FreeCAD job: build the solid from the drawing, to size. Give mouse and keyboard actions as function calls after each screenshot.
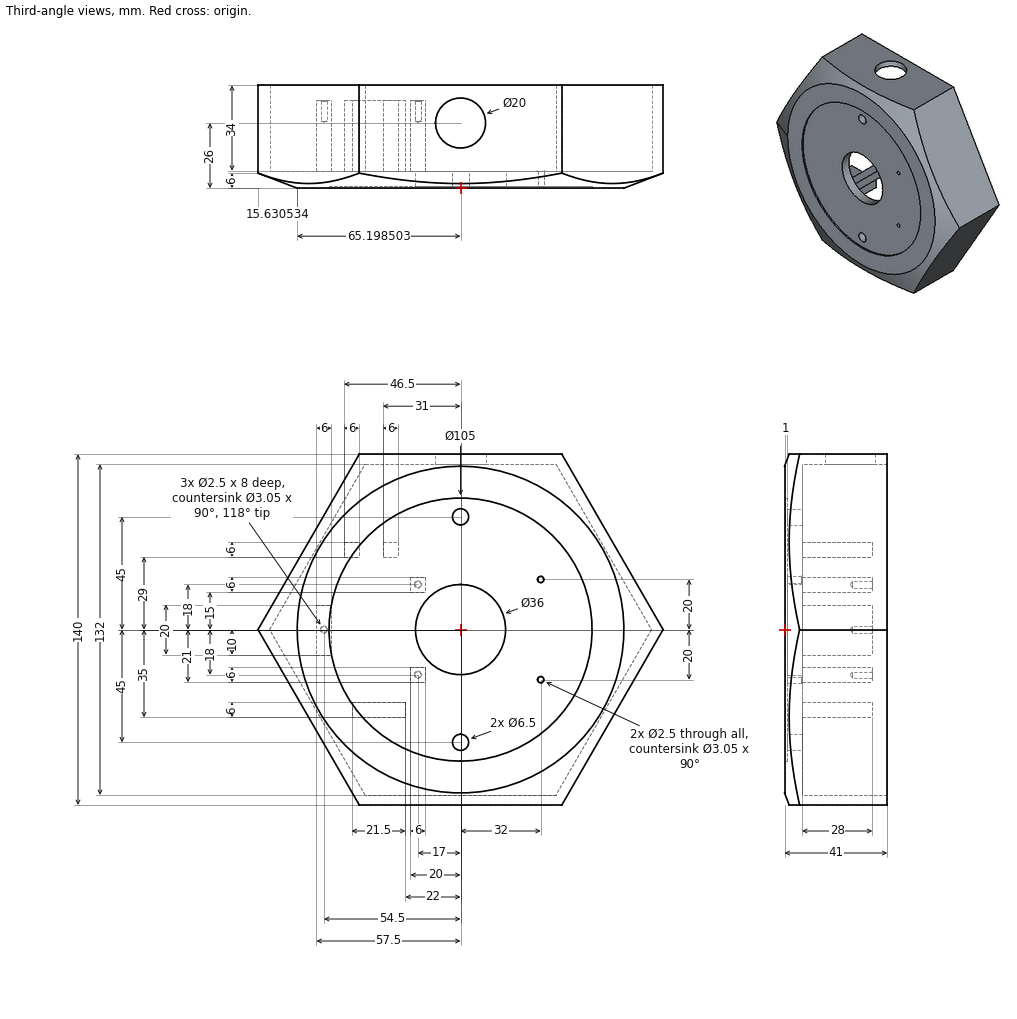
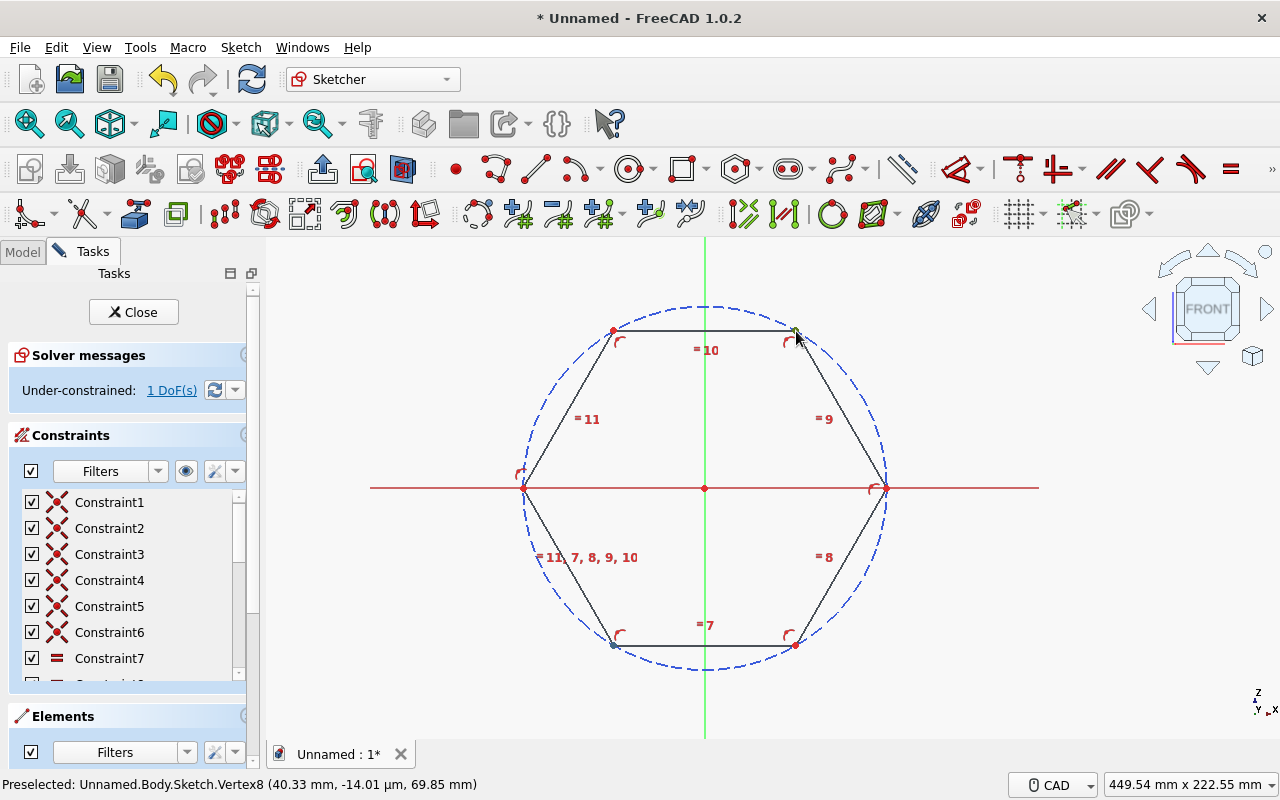
key(i)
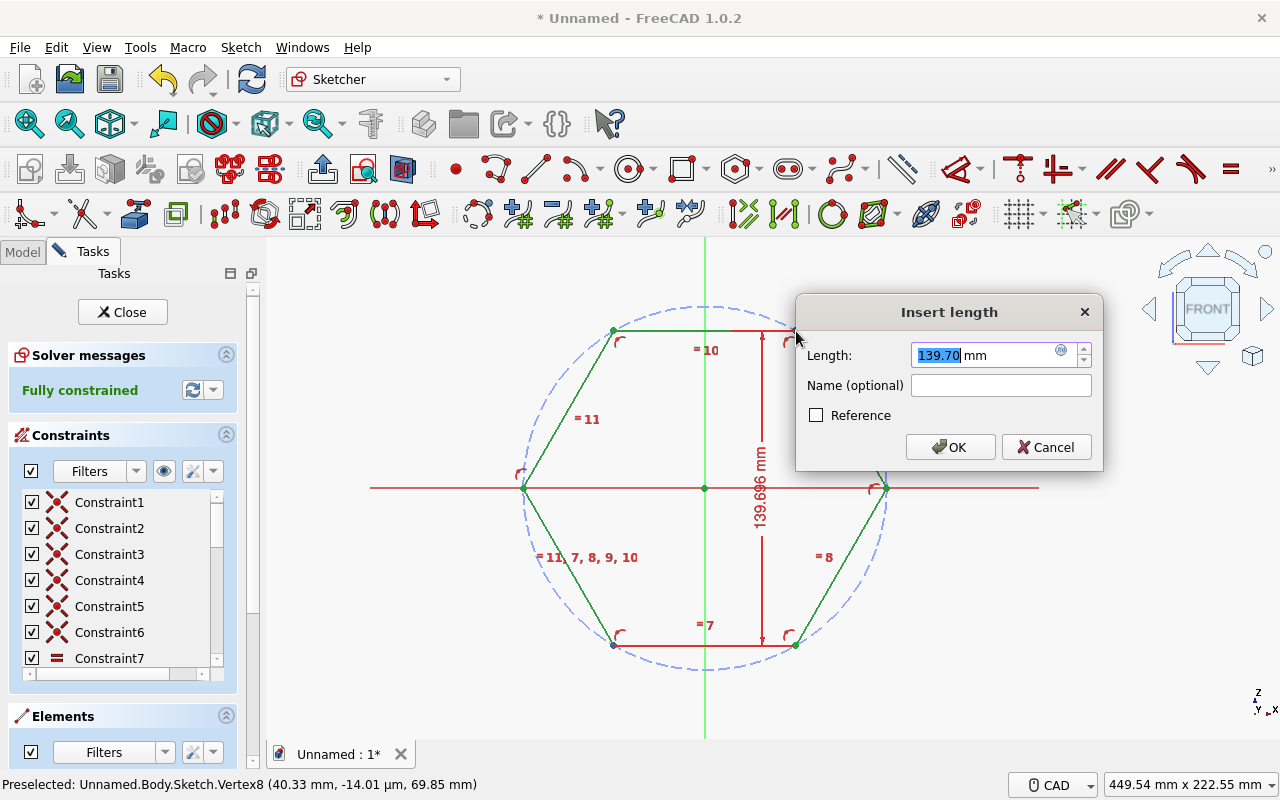
text(140)
key(Return)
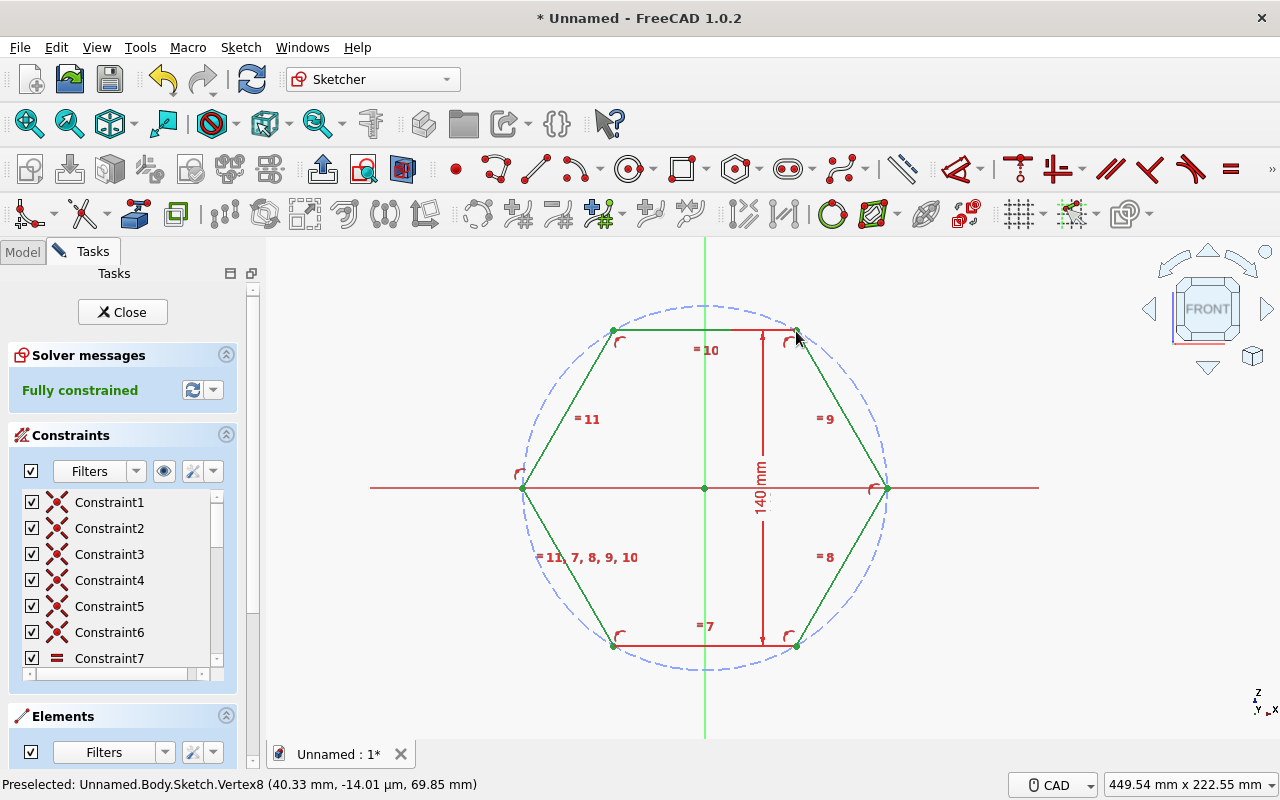
click(123, 312)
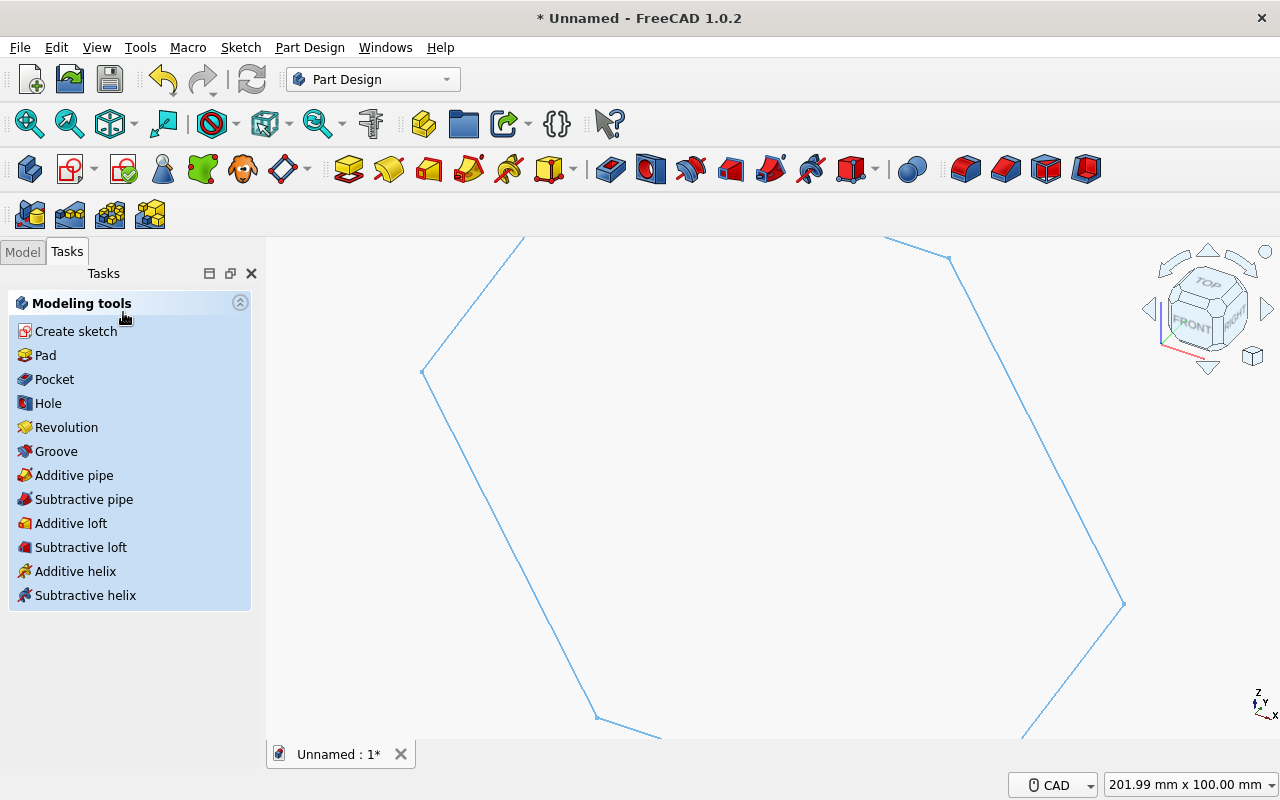
click(350, 170)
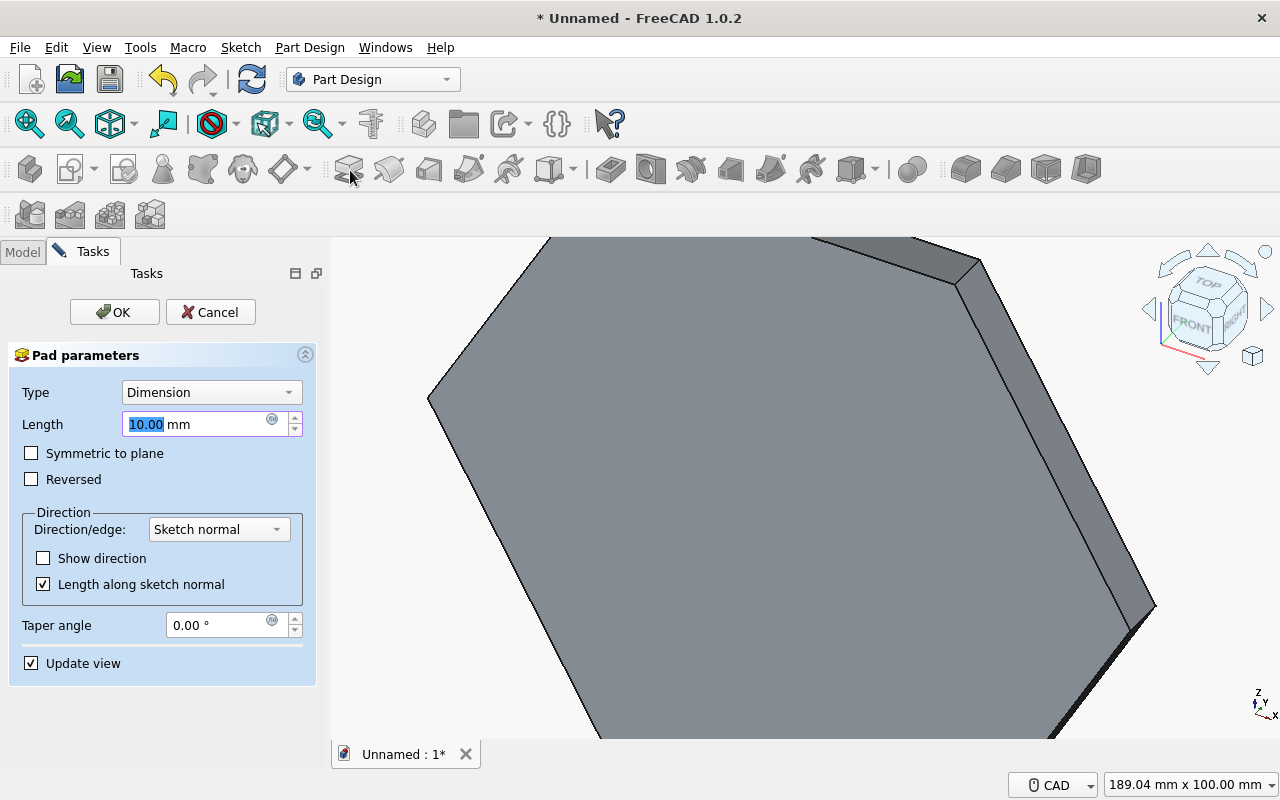
text(41)
key(Tab)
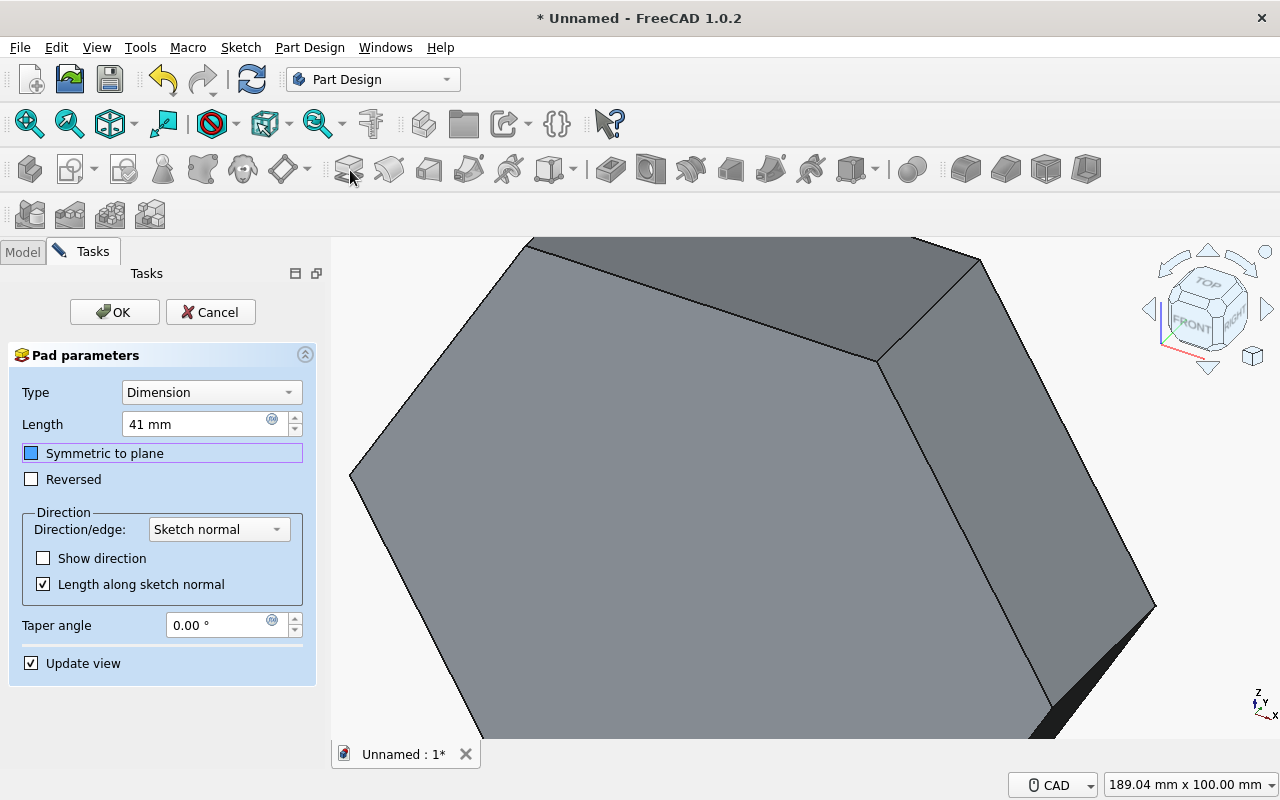
click(30, 479)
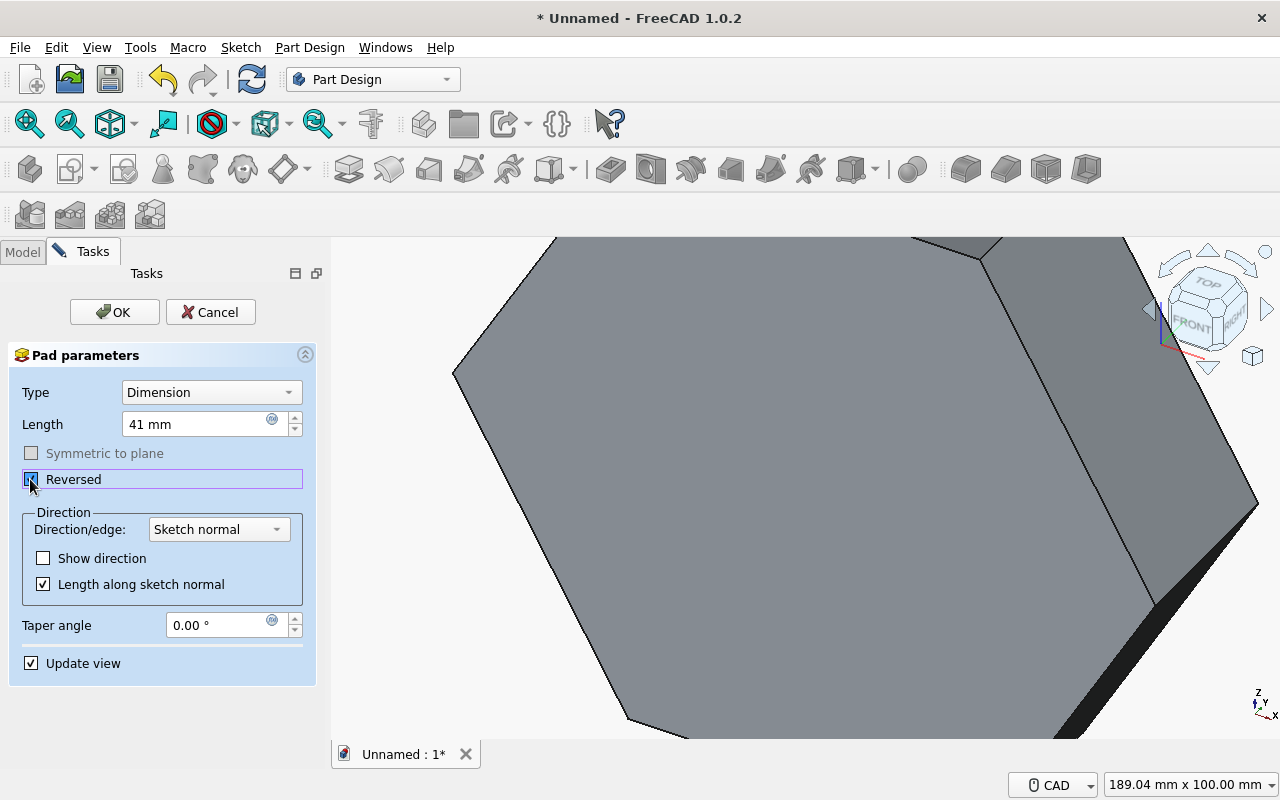
click(115, 312)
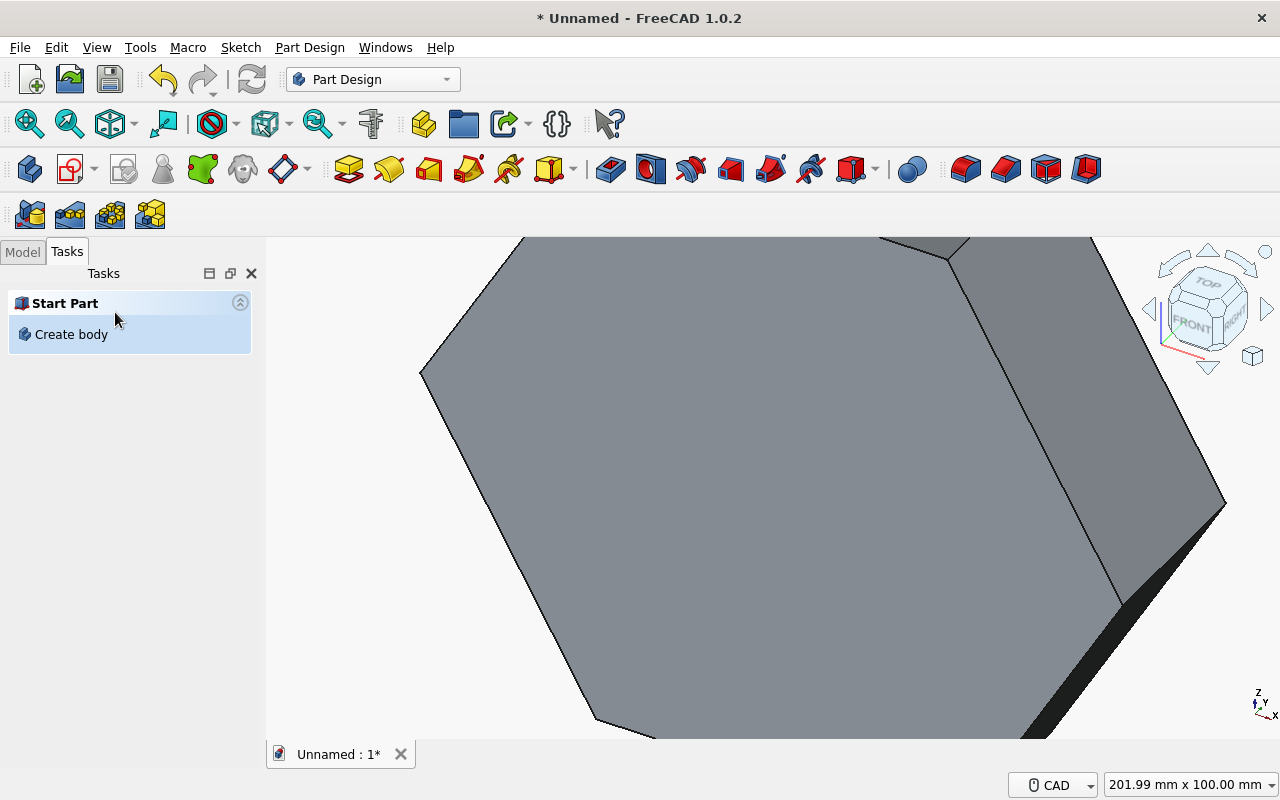
key(v)
key(f)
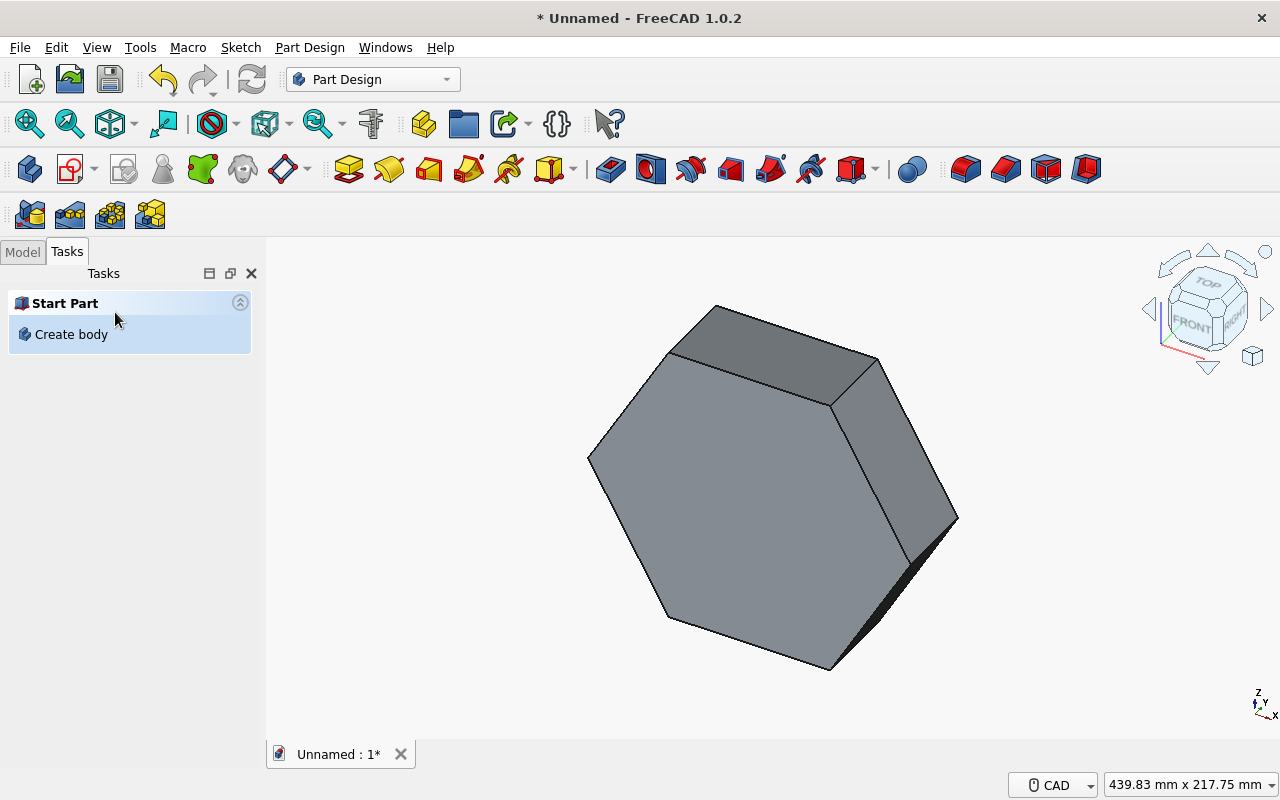
key(4)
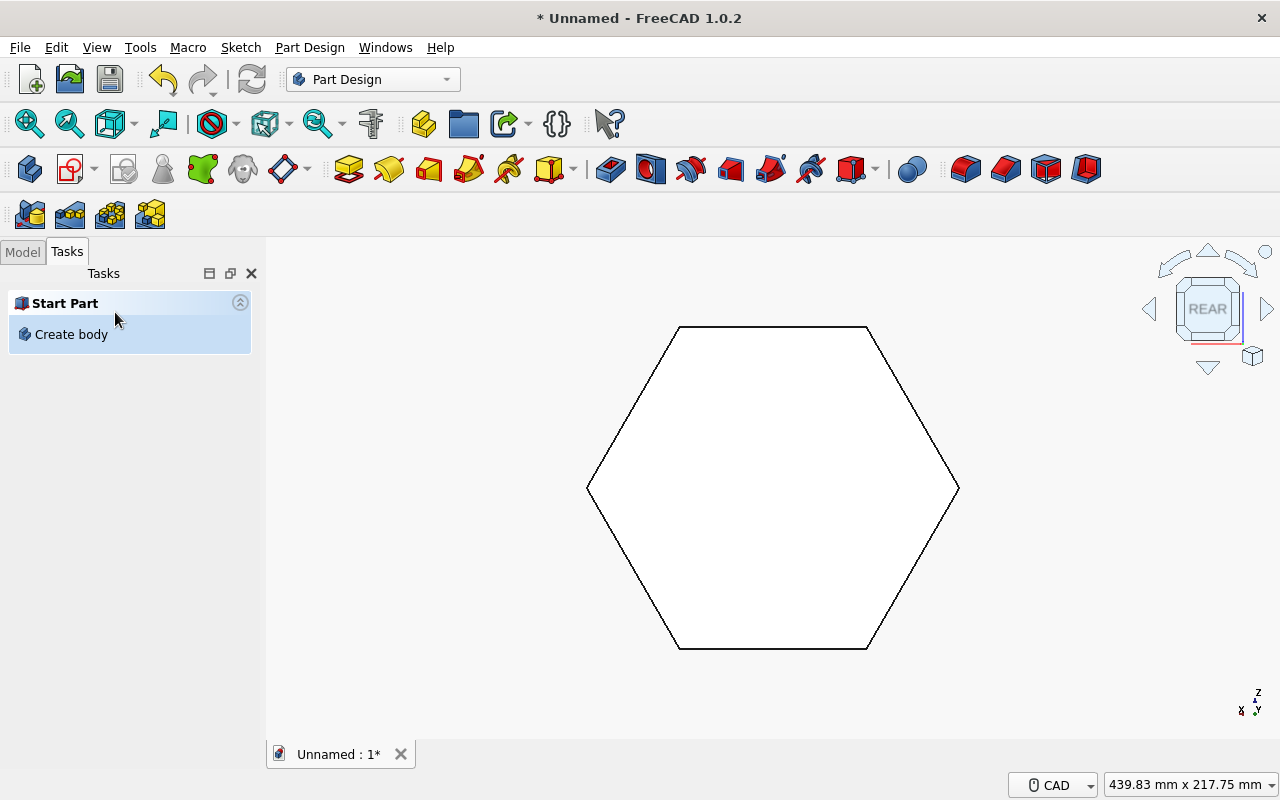
click(773, 487)